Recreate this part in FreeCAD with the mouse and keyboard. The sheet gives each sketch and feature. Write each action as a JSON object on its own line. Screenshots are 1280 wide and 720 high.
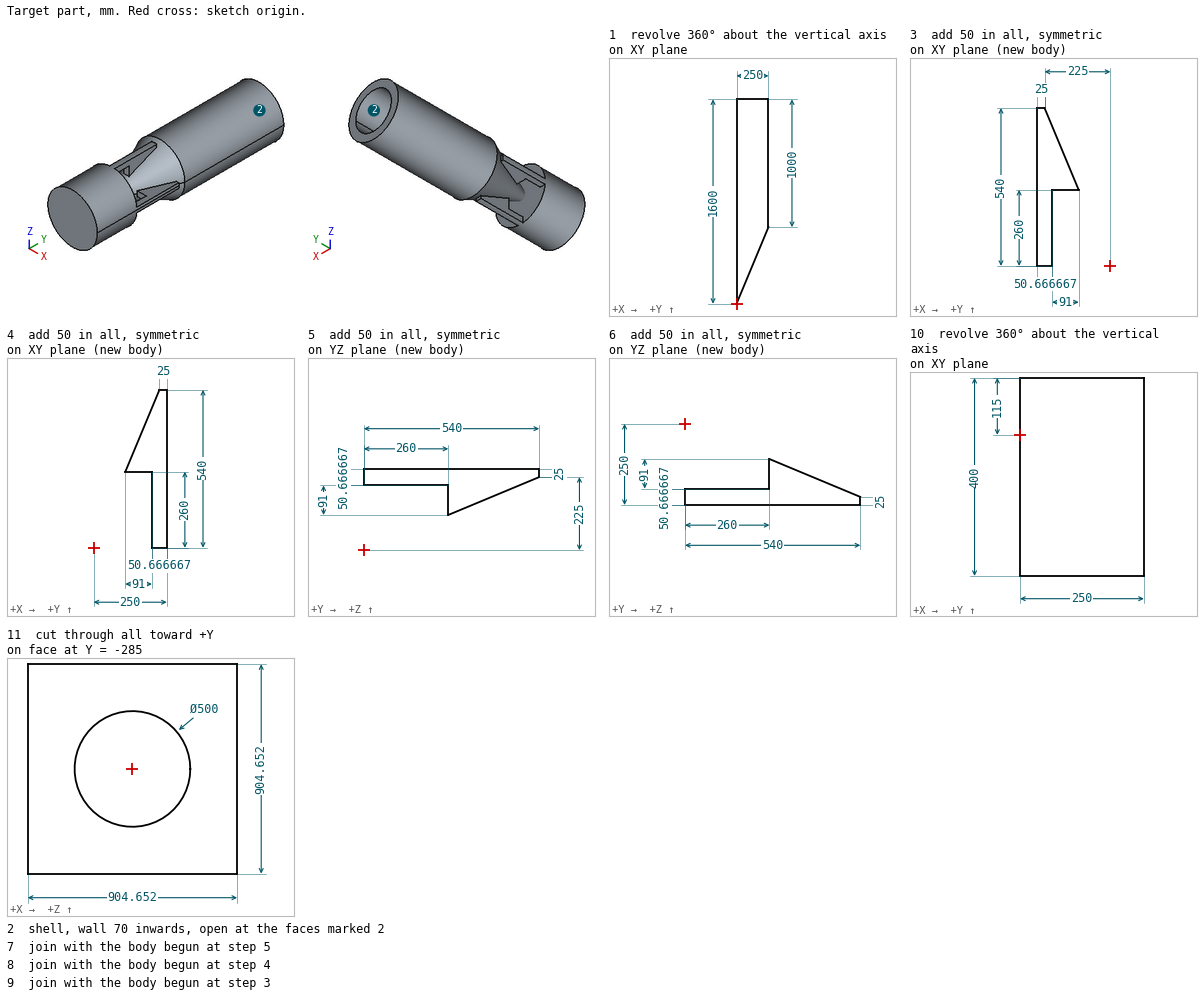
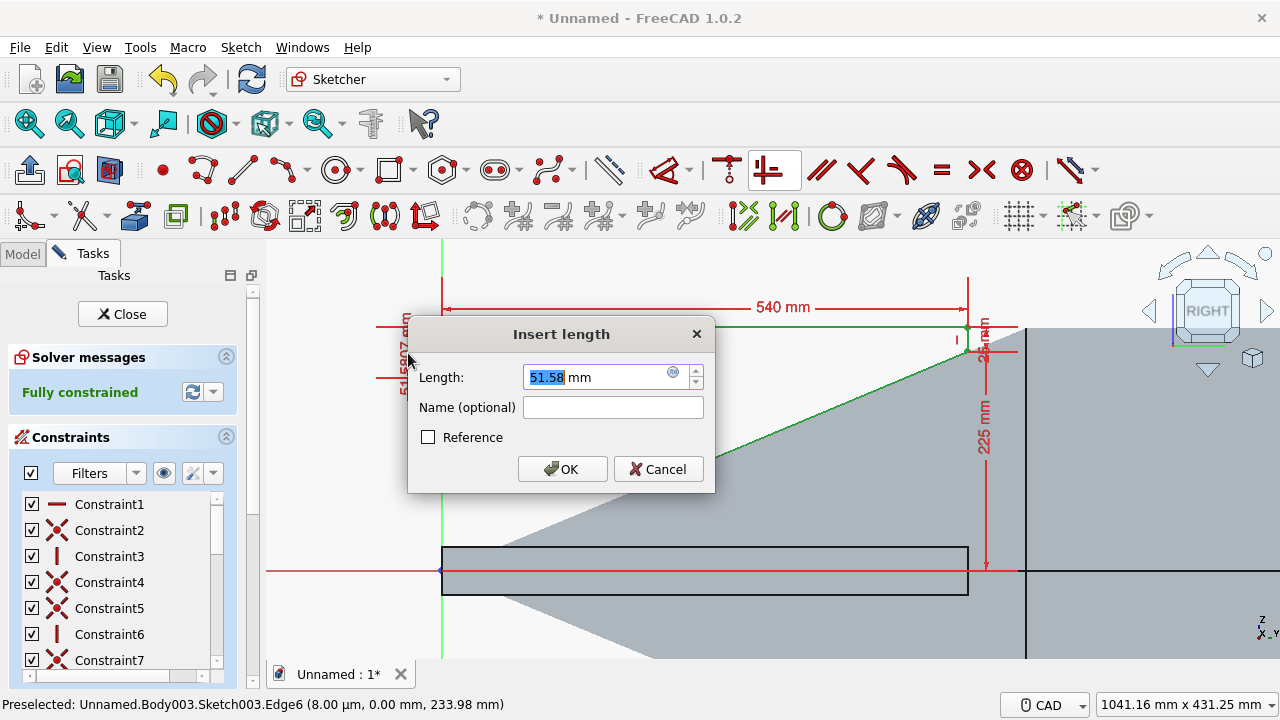
{"action": "type", "text": "50.666667"}
{"action": "key", "text": "Return"}
{"action": "key", "text": "Escape"}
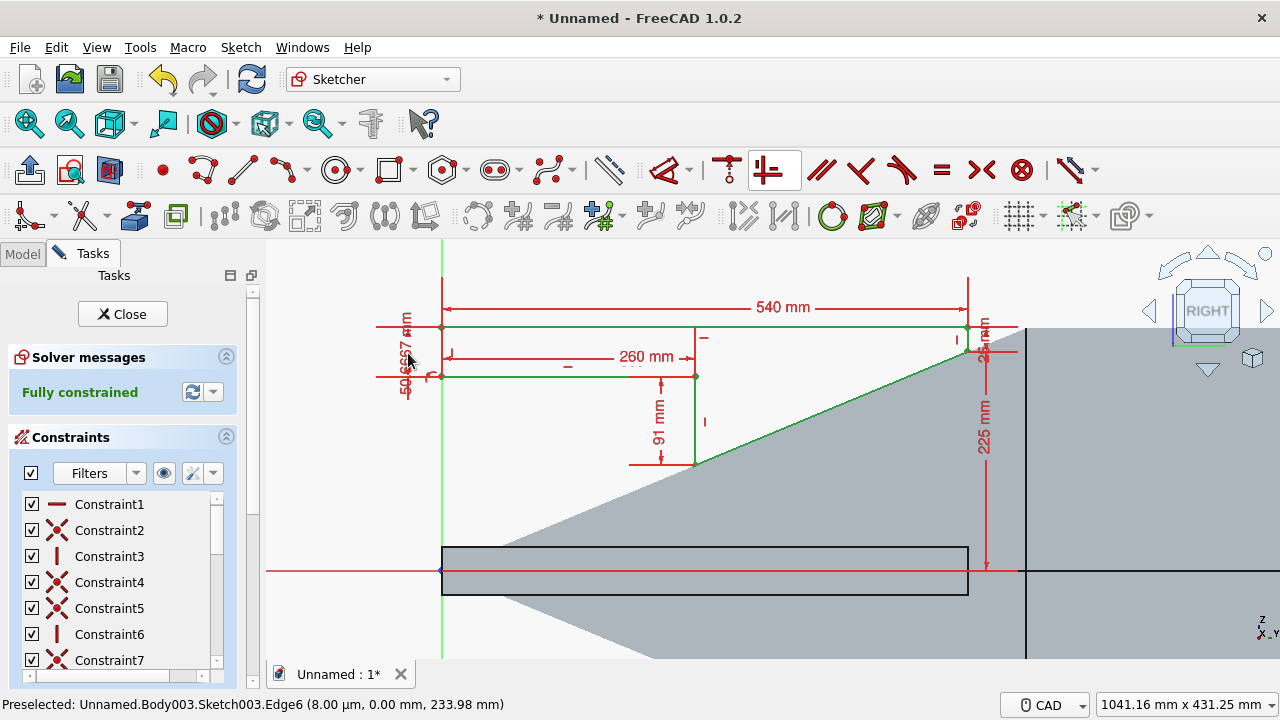
{"action": "left_click", "coordinate": [123, 314]}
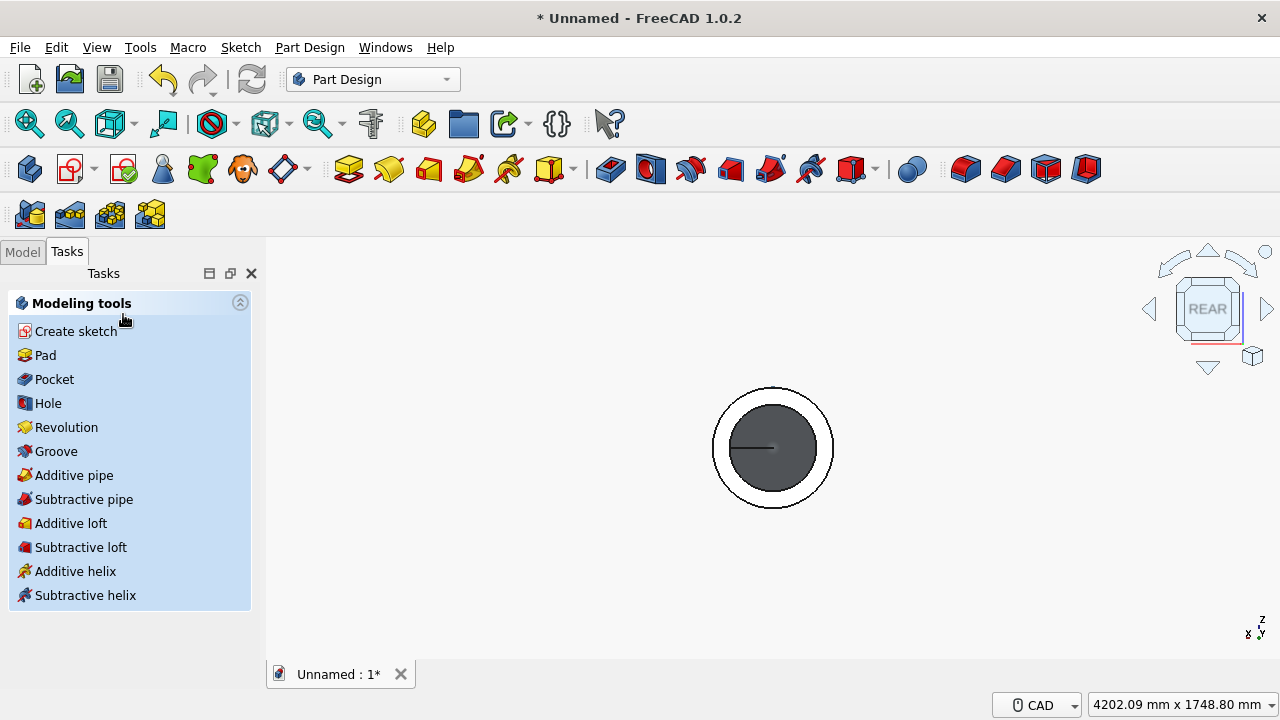
{"action": "left_click", "coordinate": [350, 170]}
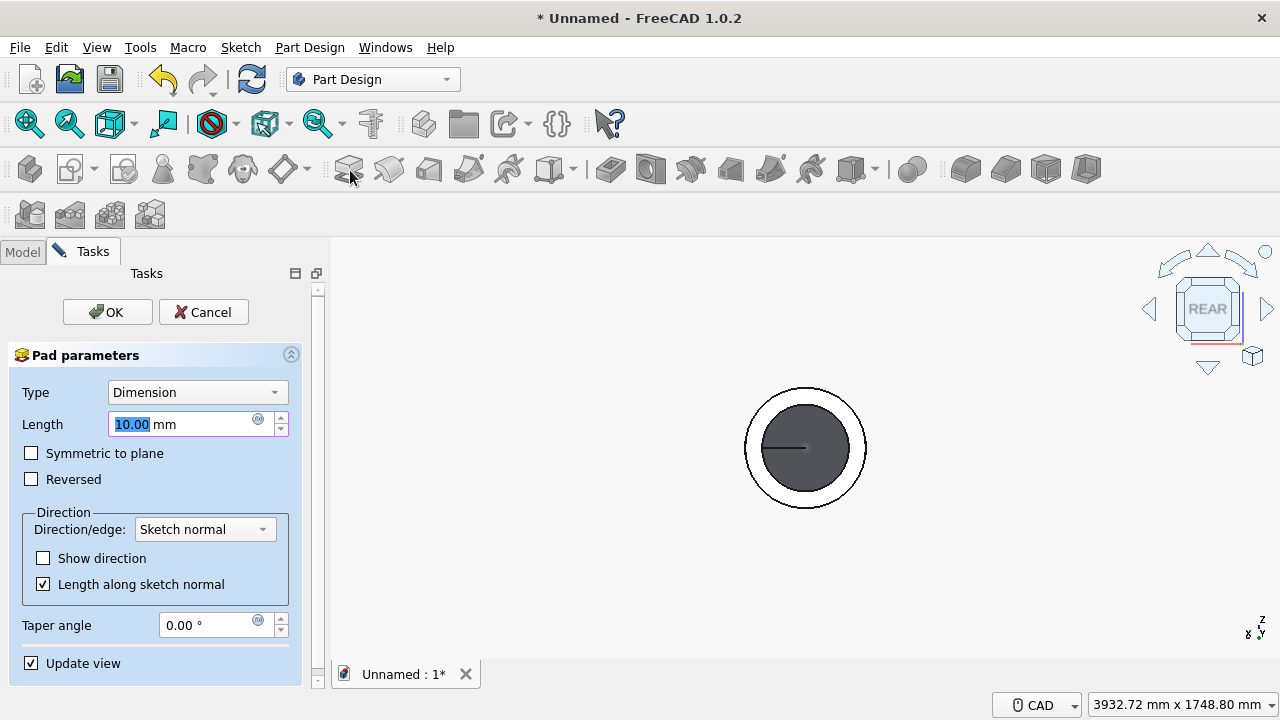
{"action": "type", "text": "50"}
{"action": "key", "text": "Tab"}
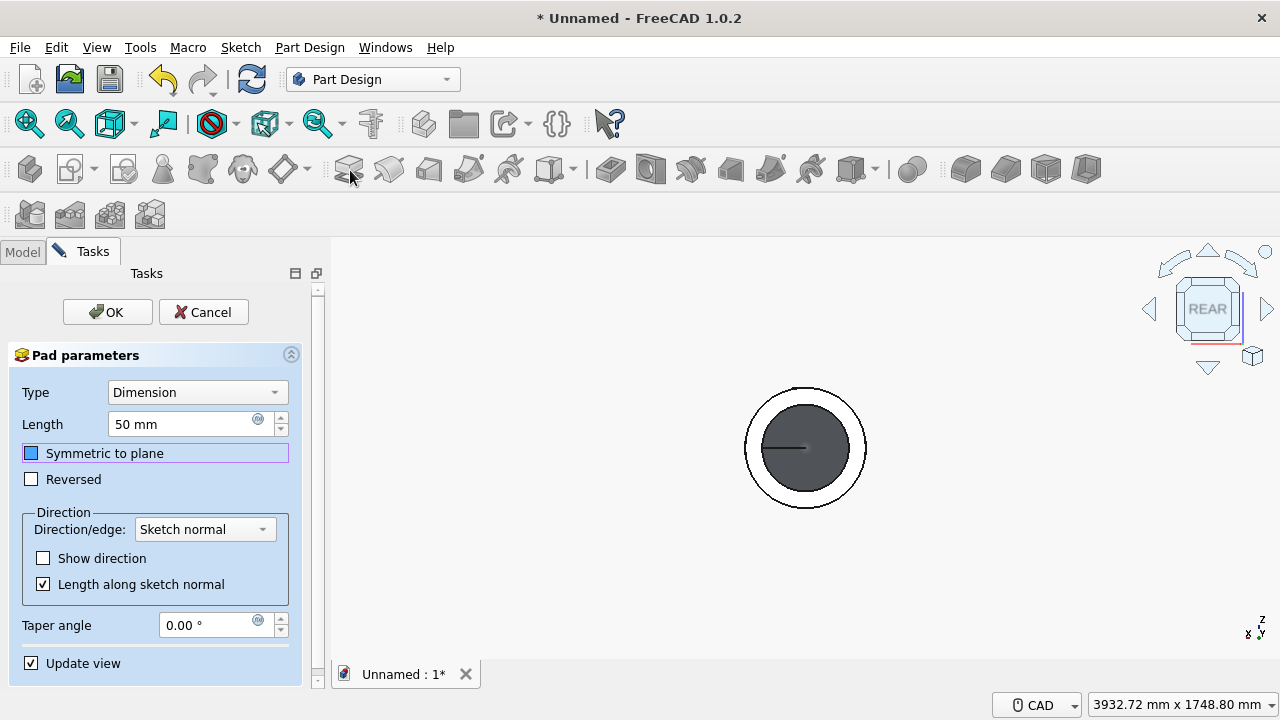
{"action": "left_click", "coordinate": [30, 453]}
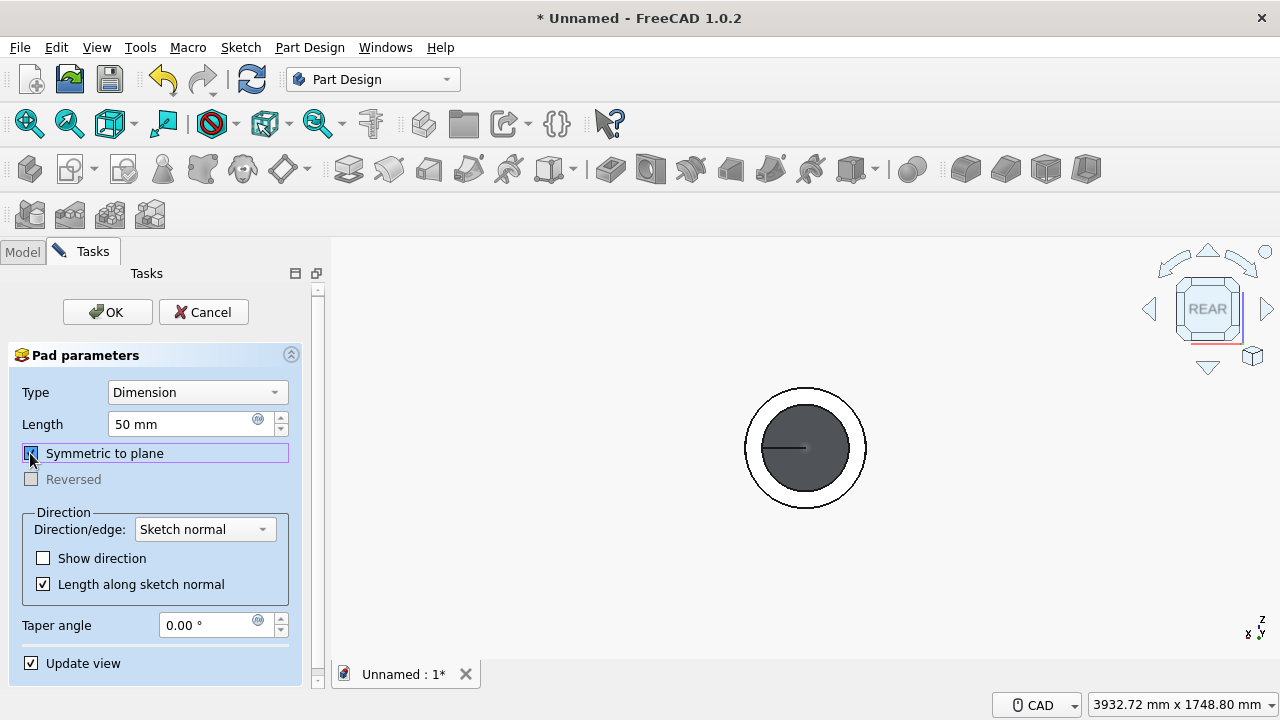
{"action": "left_click", "coordinate": [108, 312]}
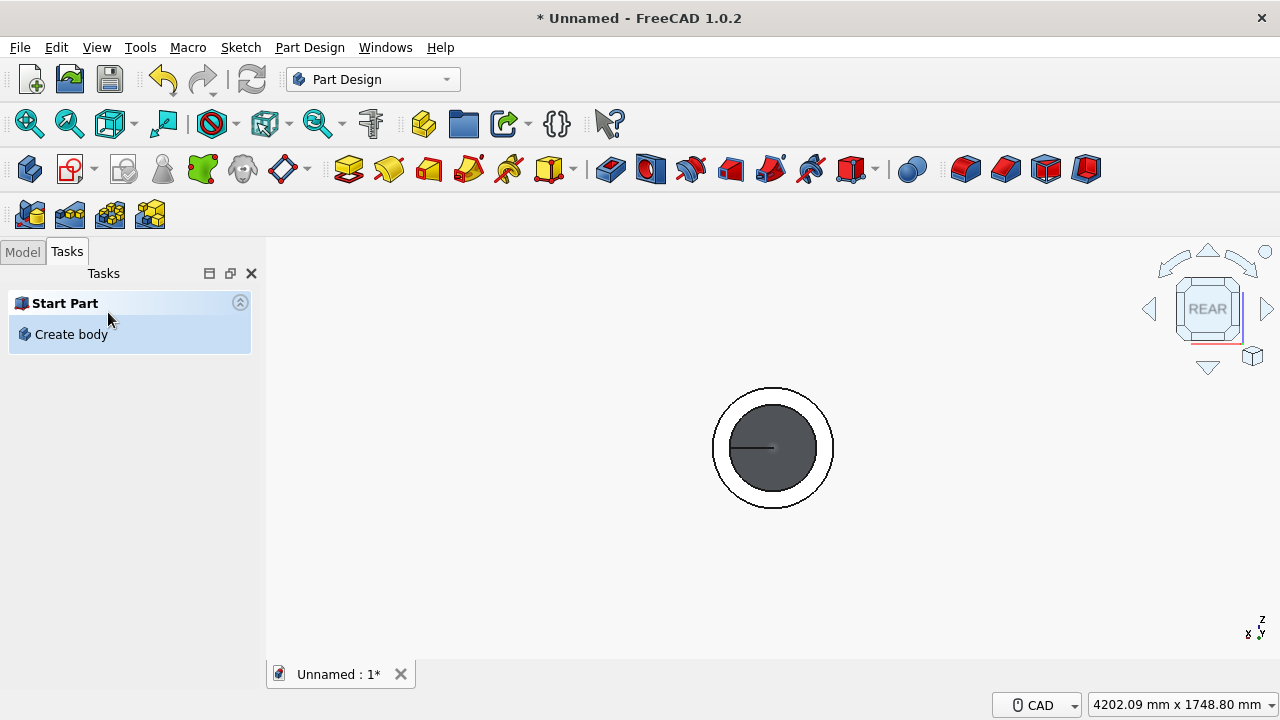
{"action": "left_click", "coordinate": [30, 124]}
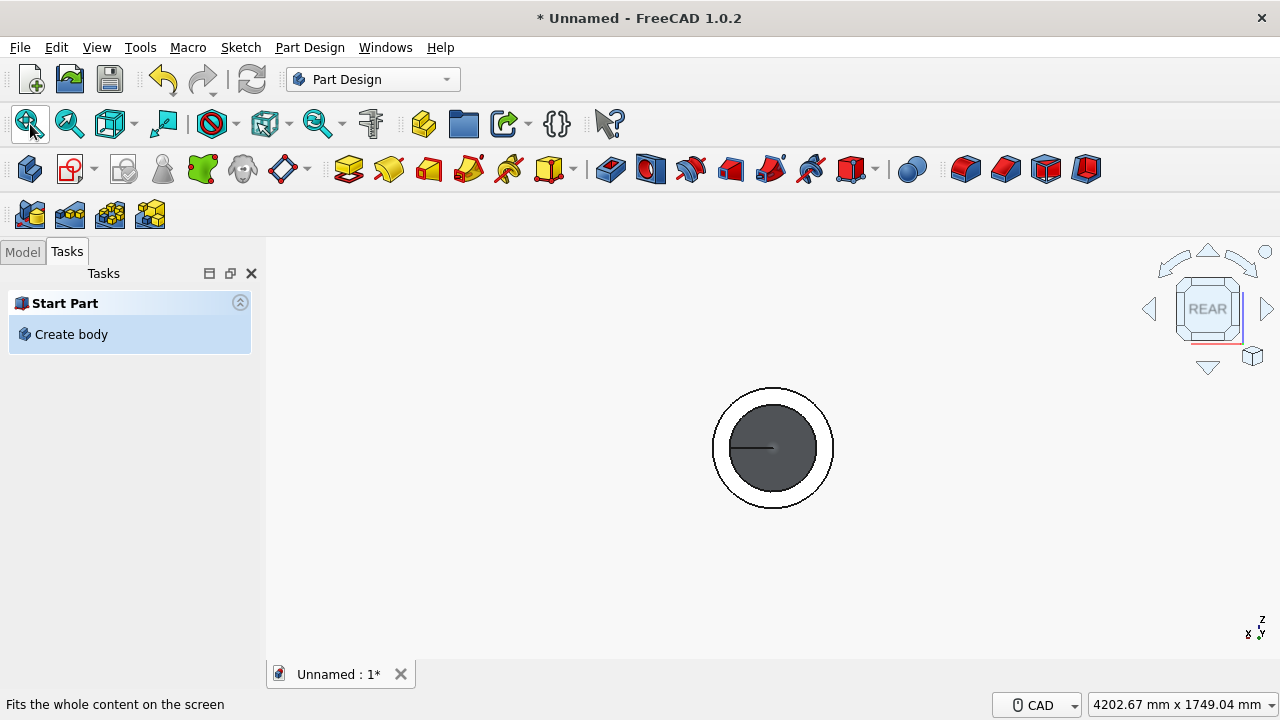
{"action": "left_click", "coordinate": [30, 170]}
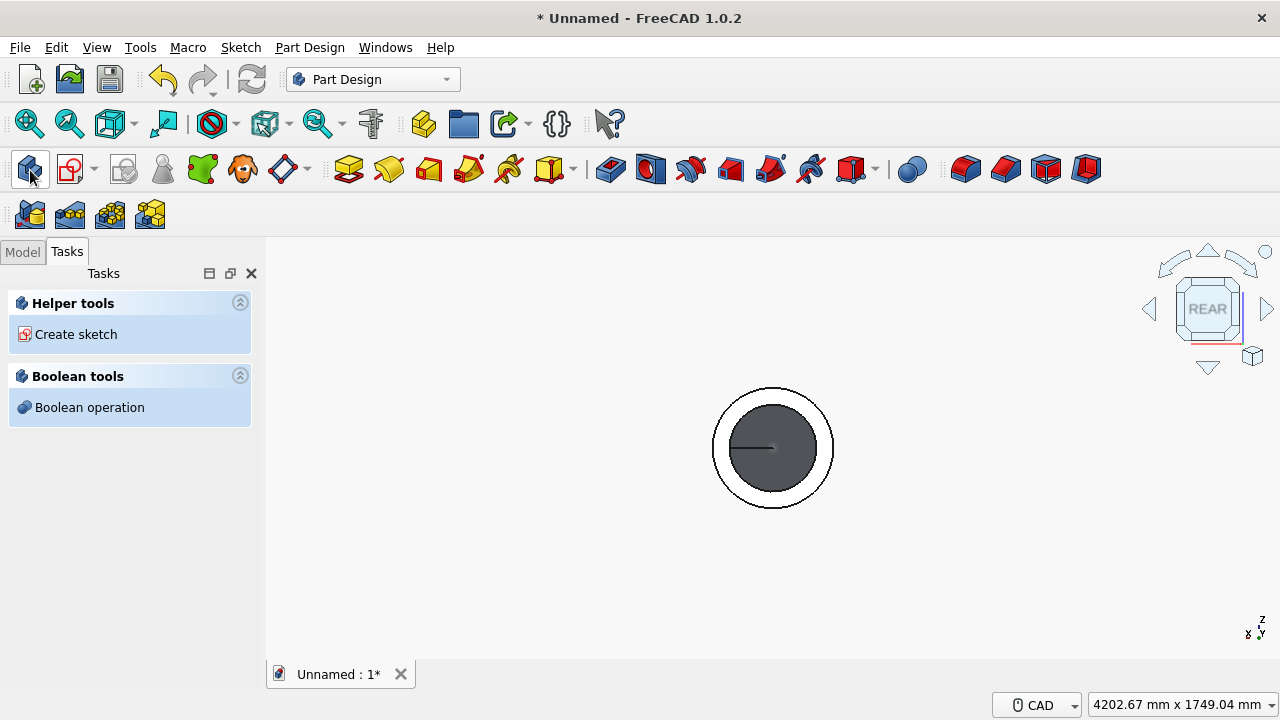
{"action": "left_click", "coordinate": [306, 619]}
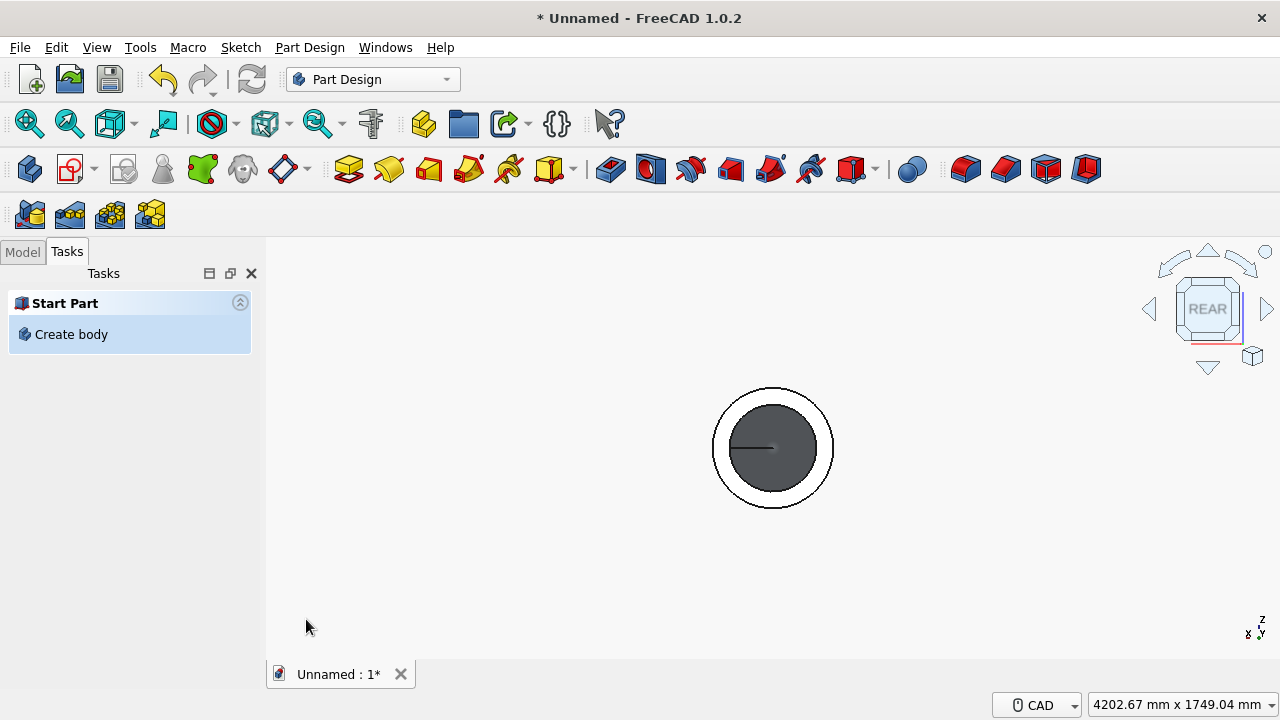
{"action": "left_click", "coordinate": [70, 170]}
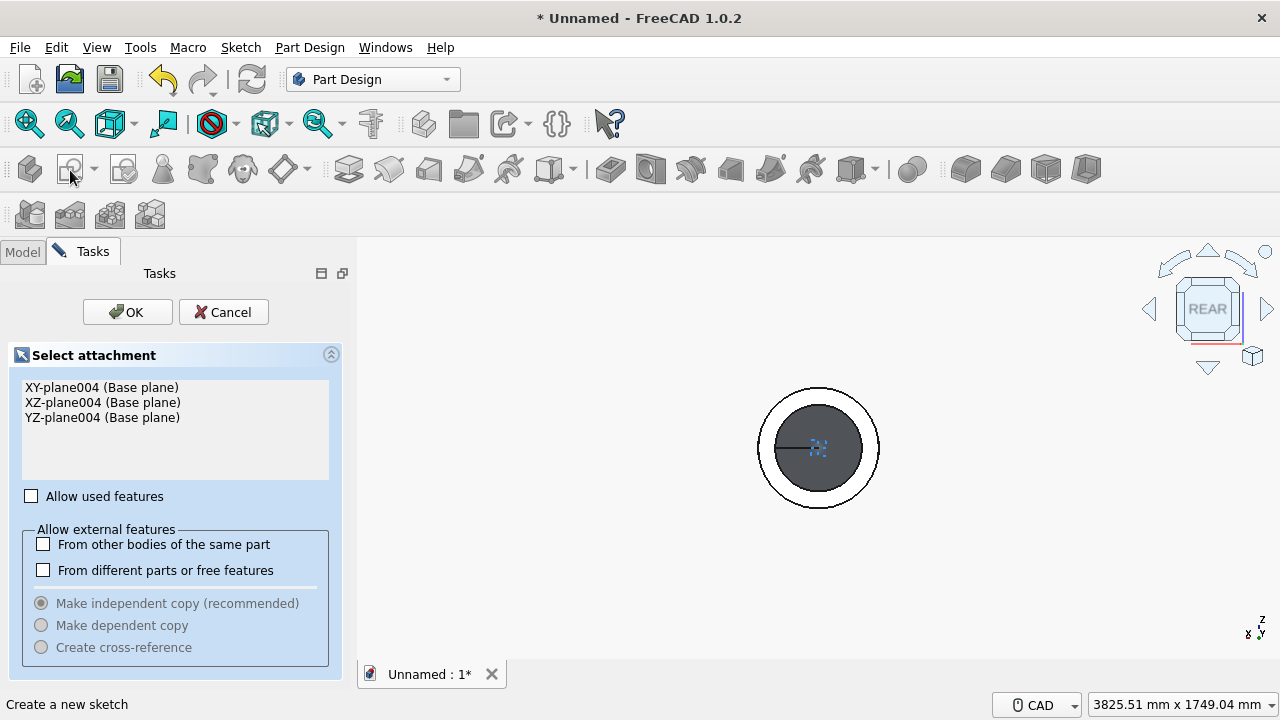
{"action": "left_click", "coordinate": [82, 418]}